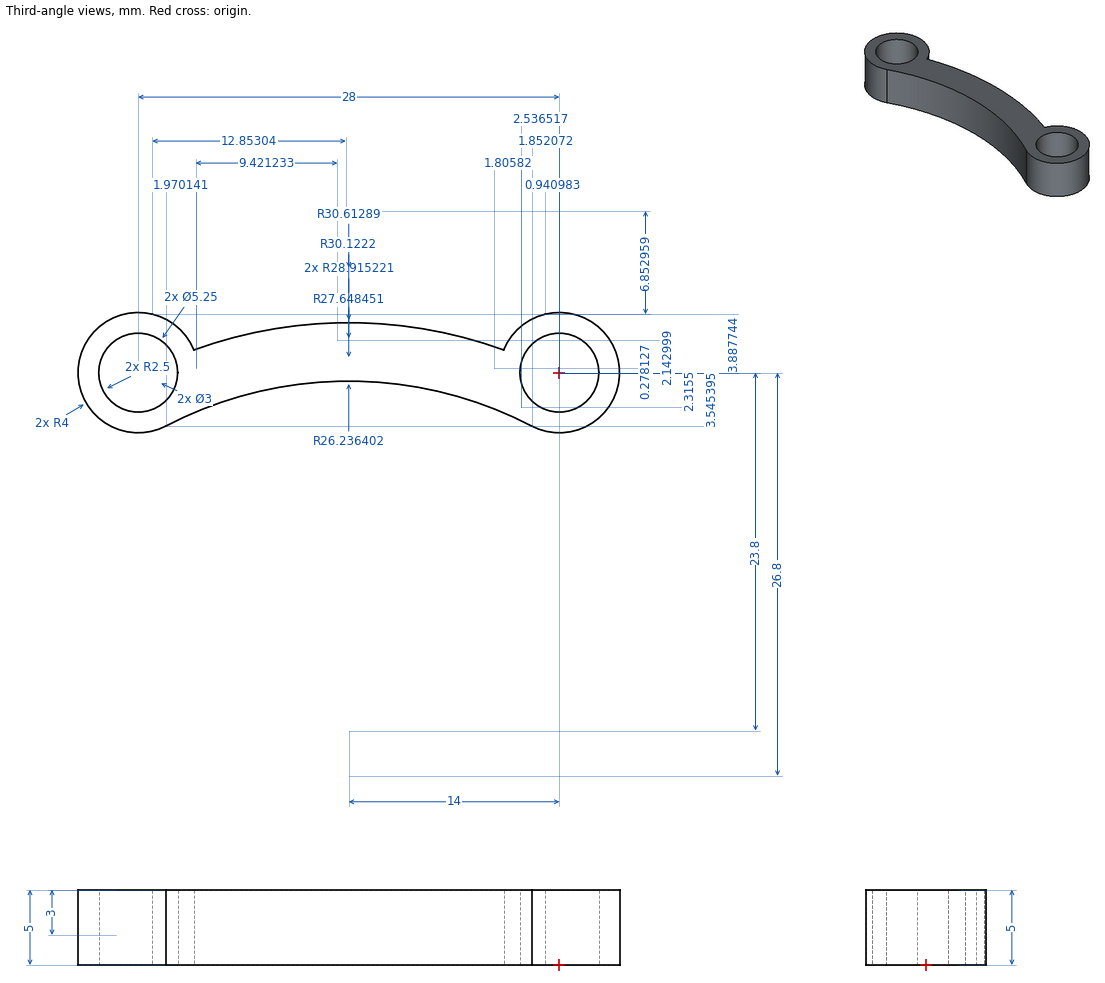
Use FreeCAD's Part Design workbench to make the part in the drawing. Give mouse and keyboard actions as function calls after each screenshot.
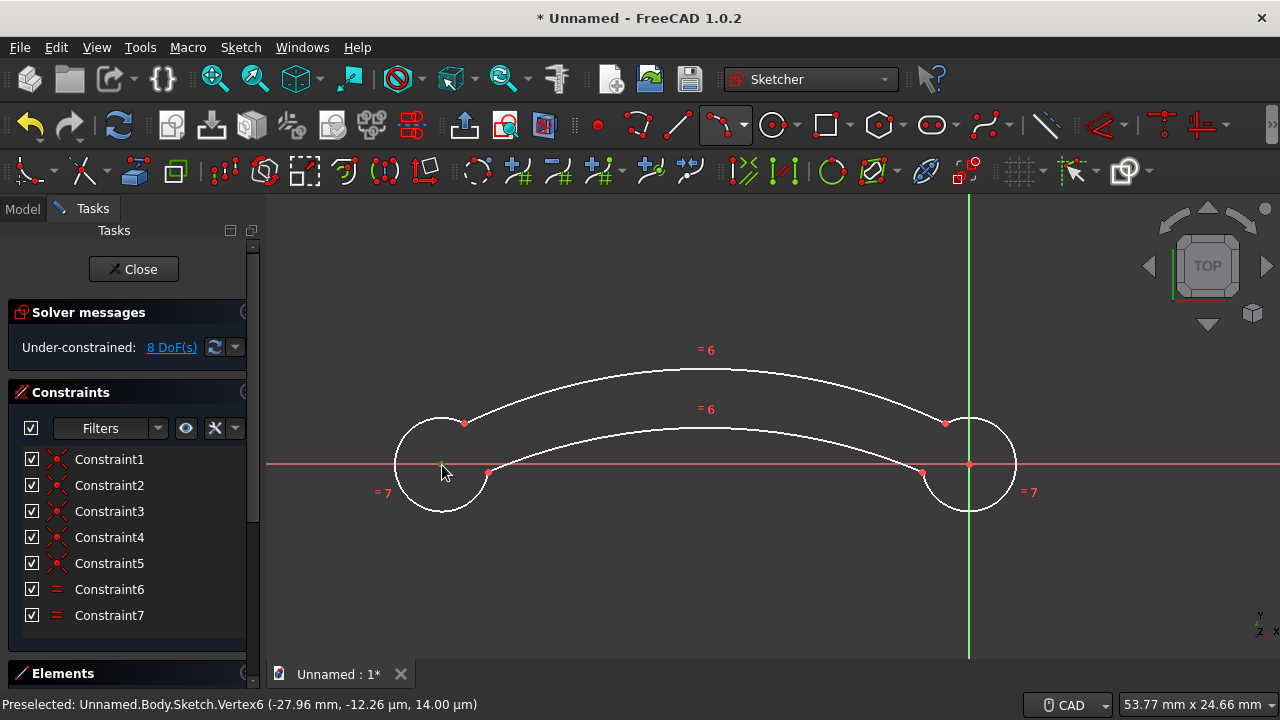
click(353, 464)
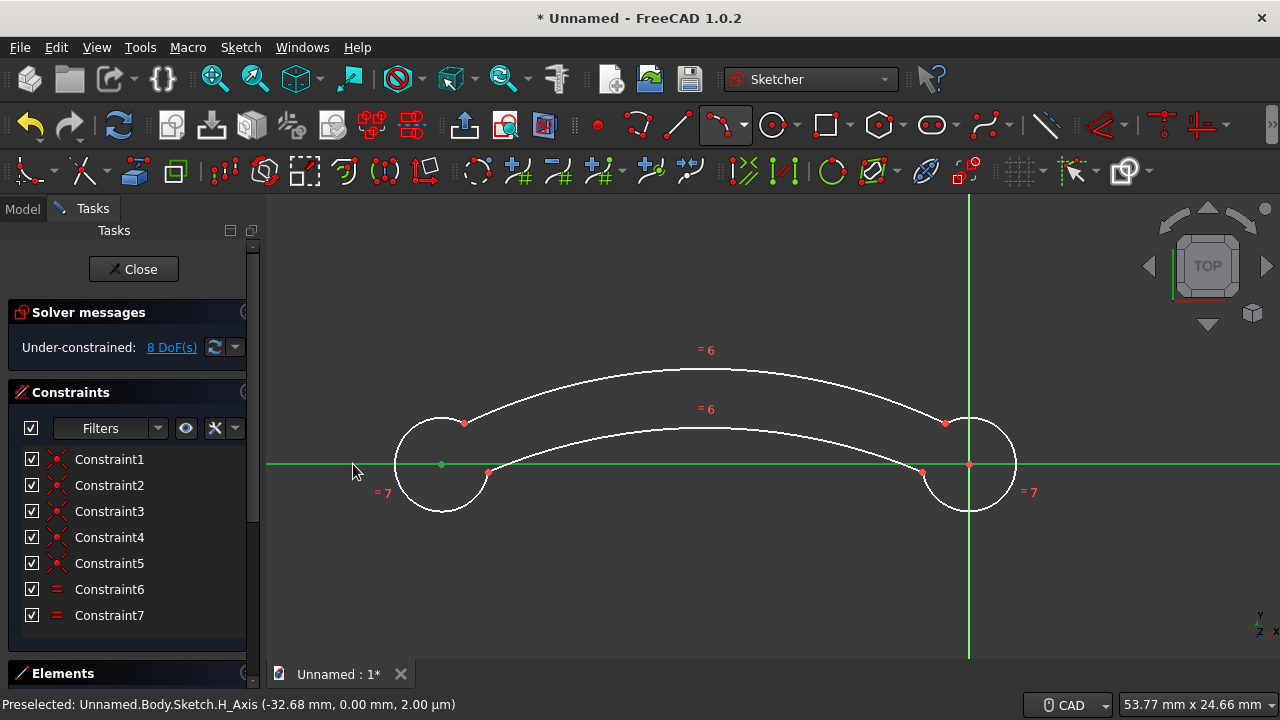
click(1162, 126)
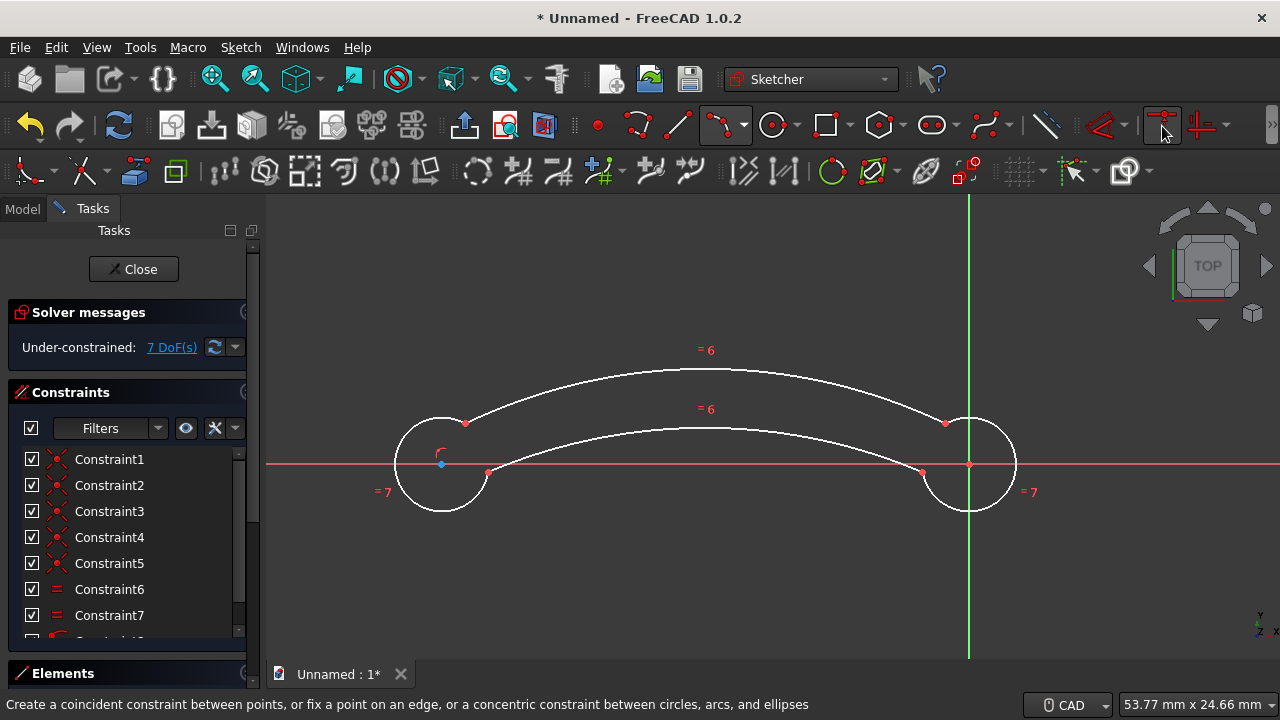
click(1100, 126)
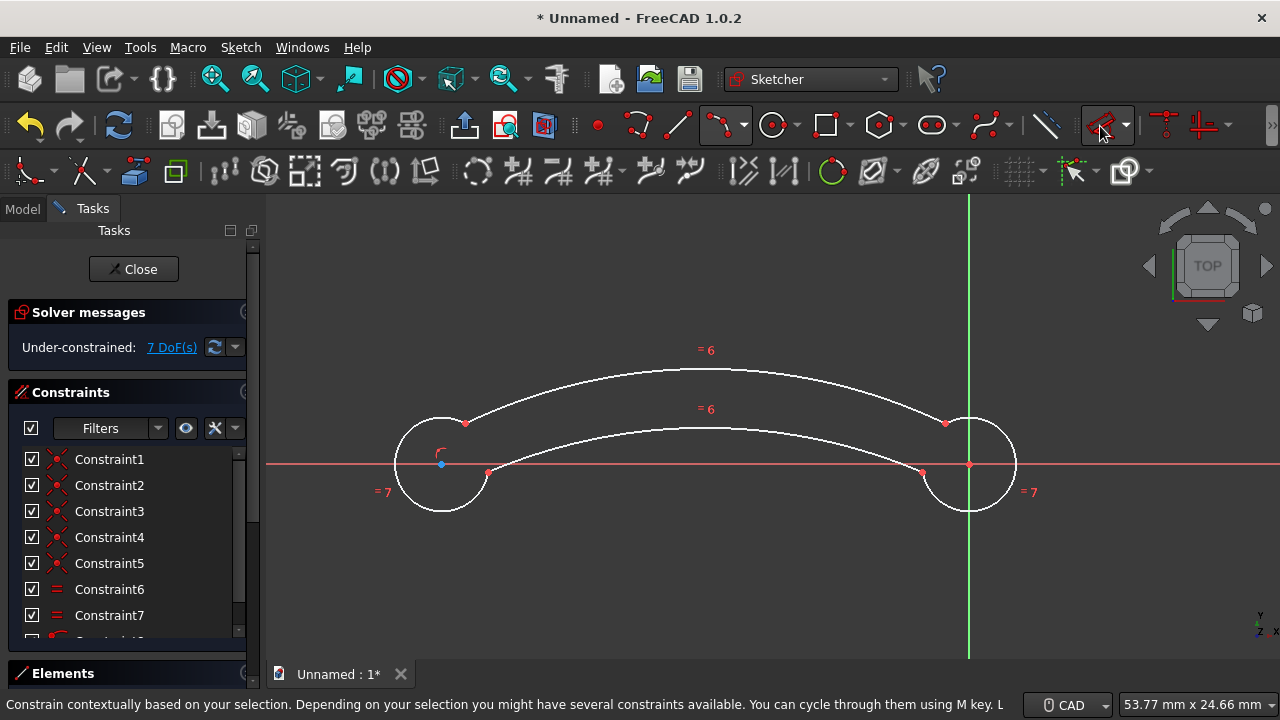
click(804, 378)
click(810, 347)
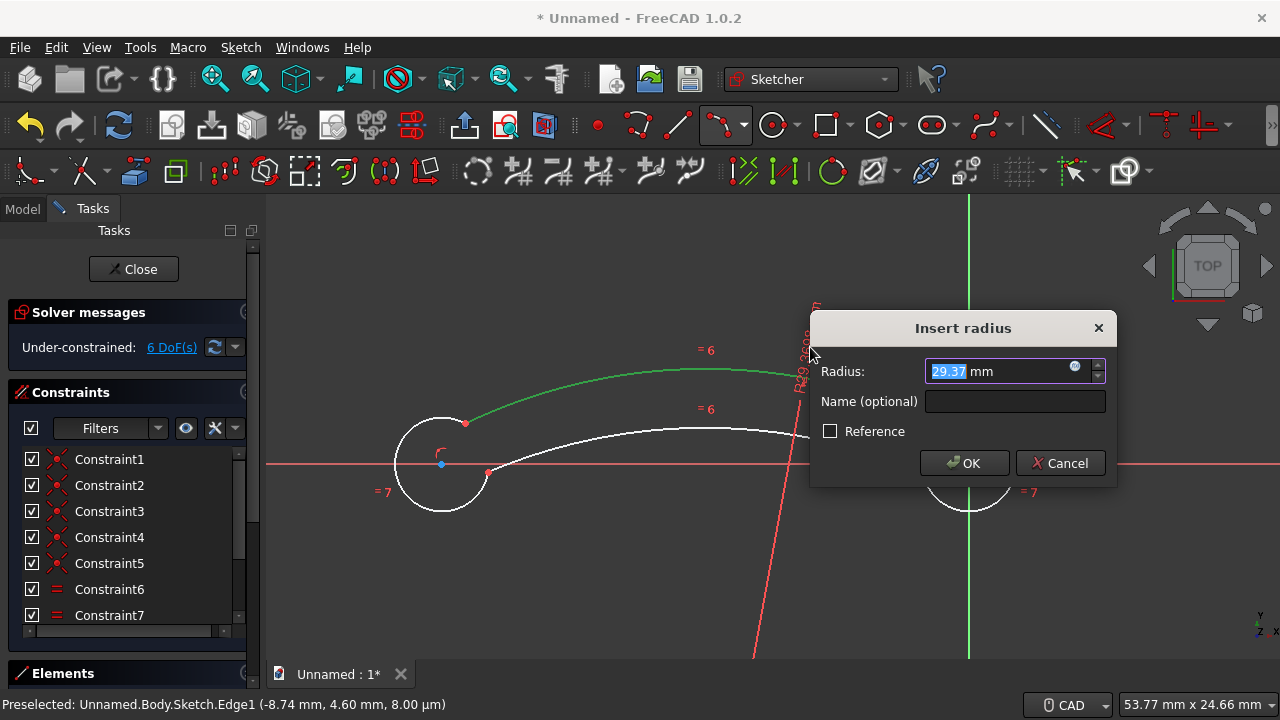
text(28.915221)
key(Return)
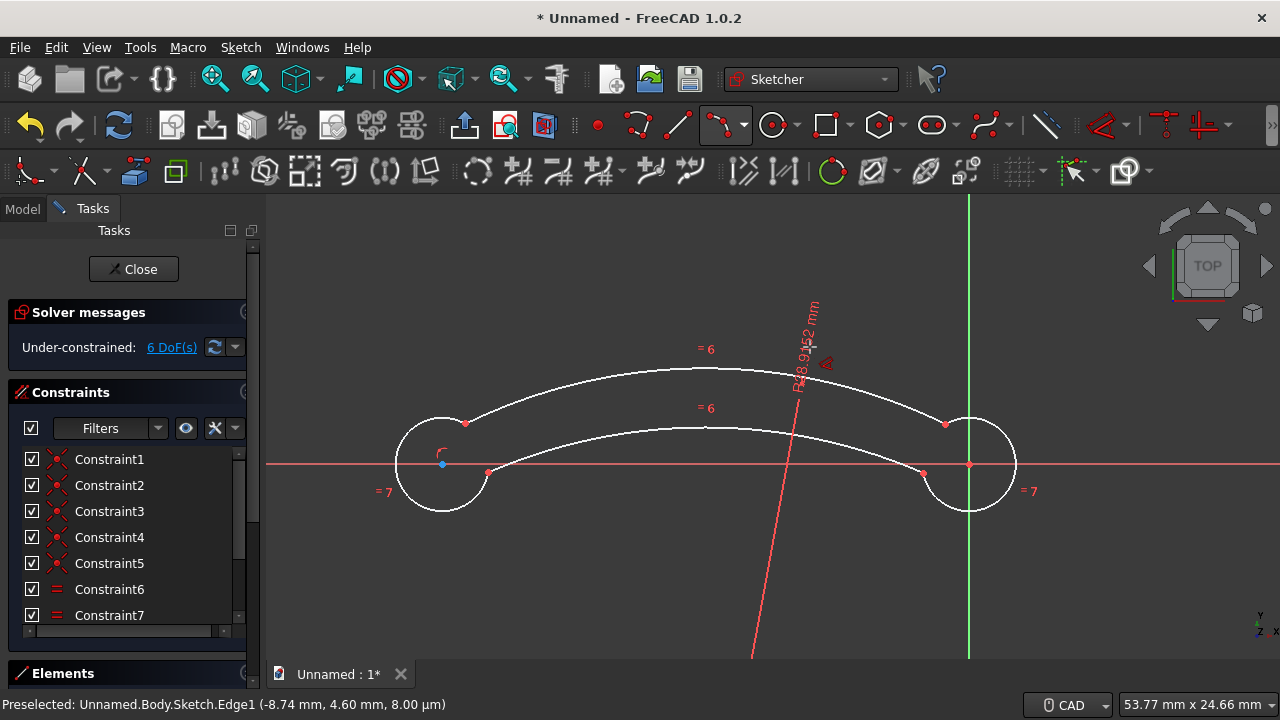
click(403, 439)
click(376, 422)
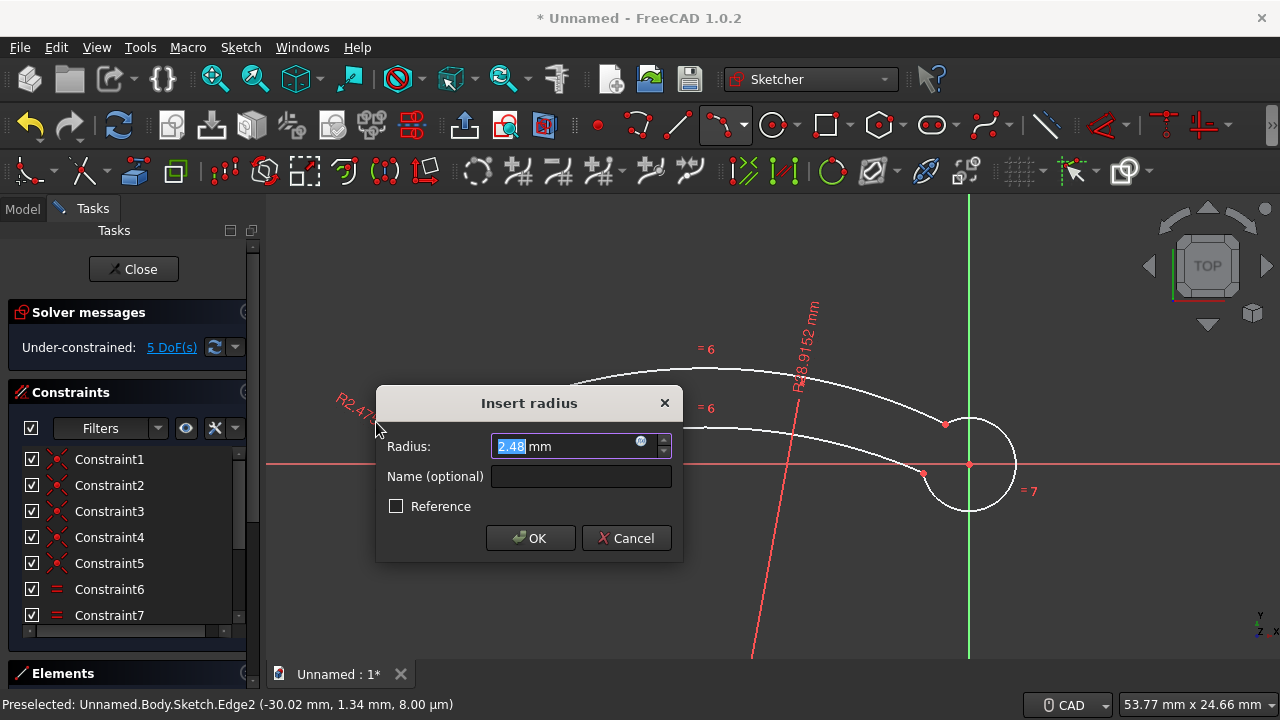
text(2.5)
key(Return)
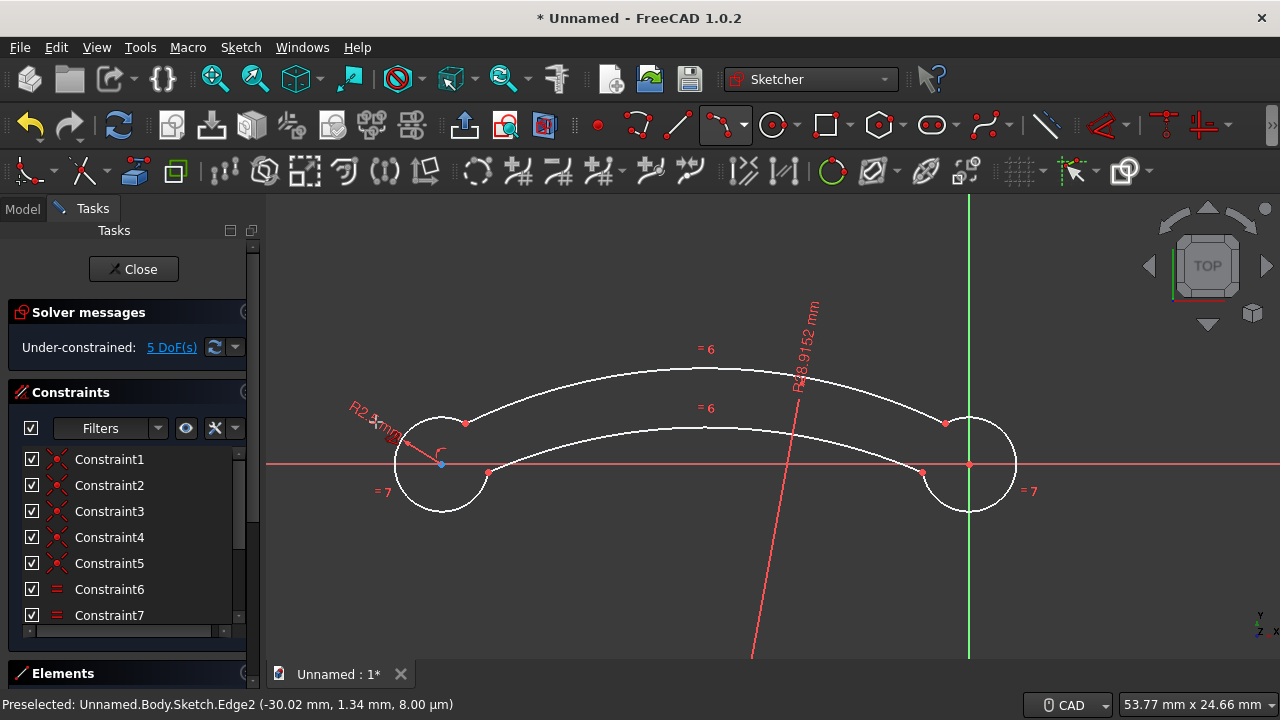
scroll(704, 222, down, 3)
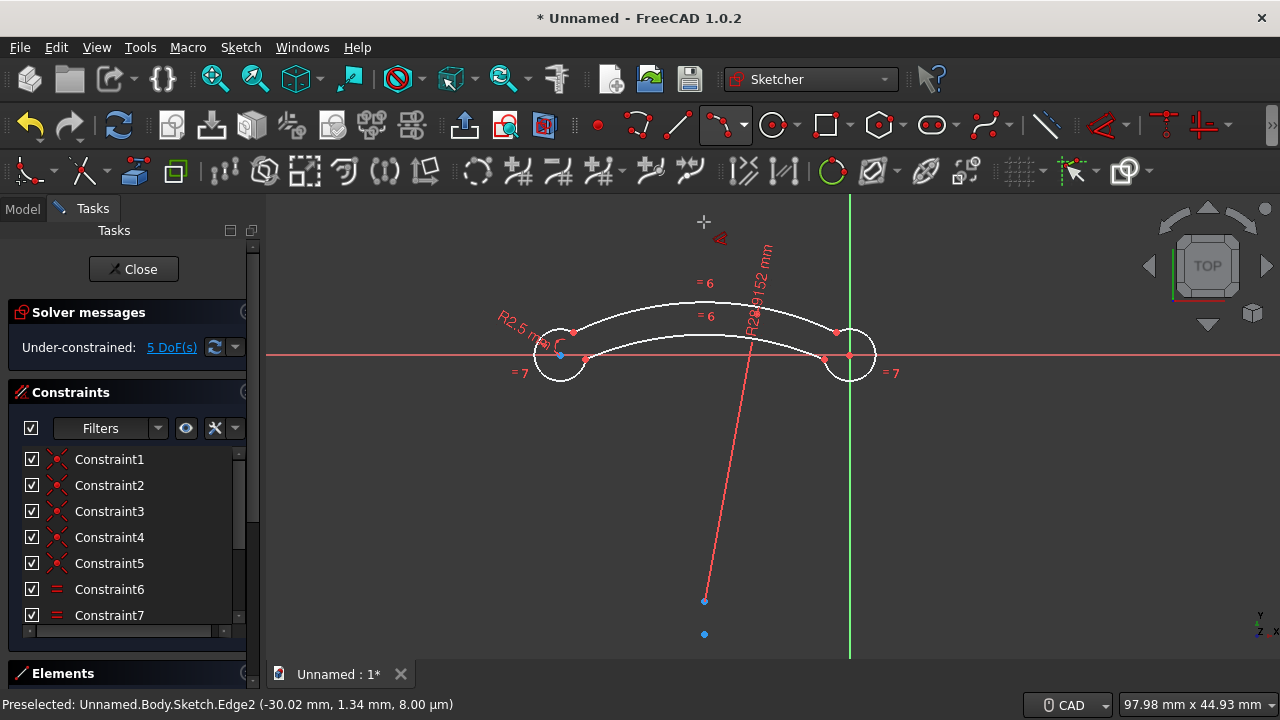
click(705, 602)
click(744, 321)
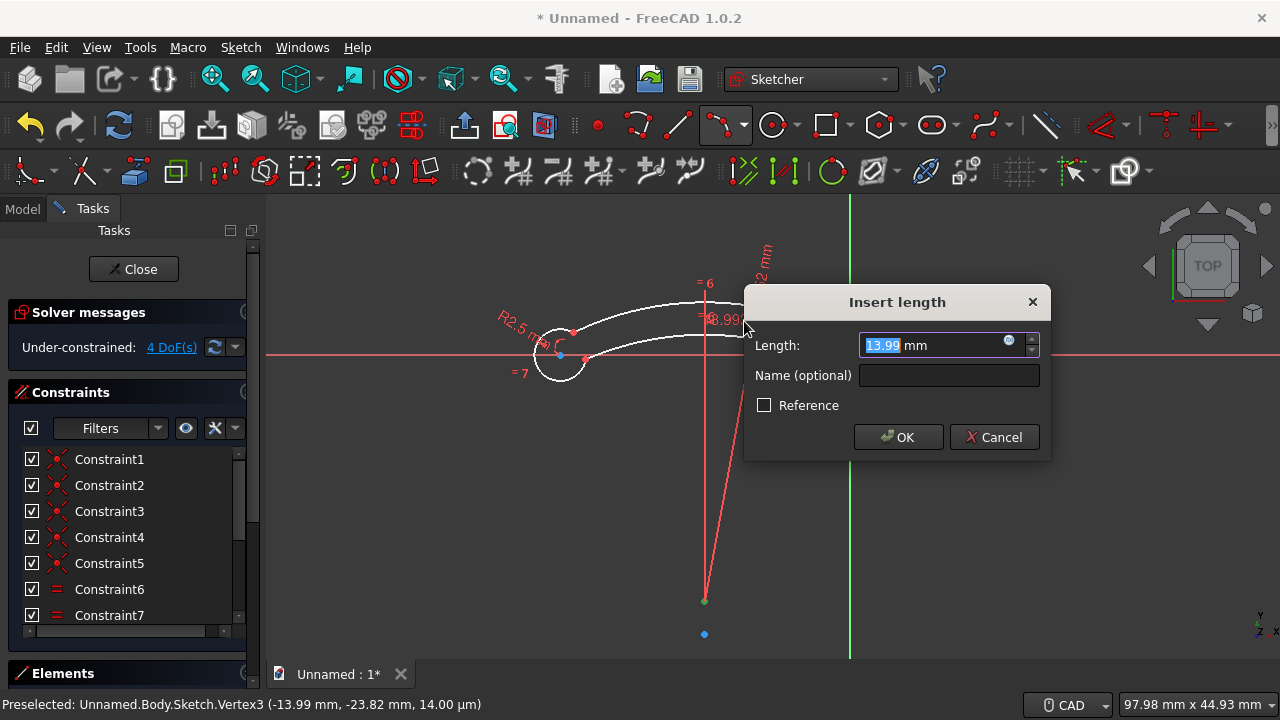
text(14)
key(Return)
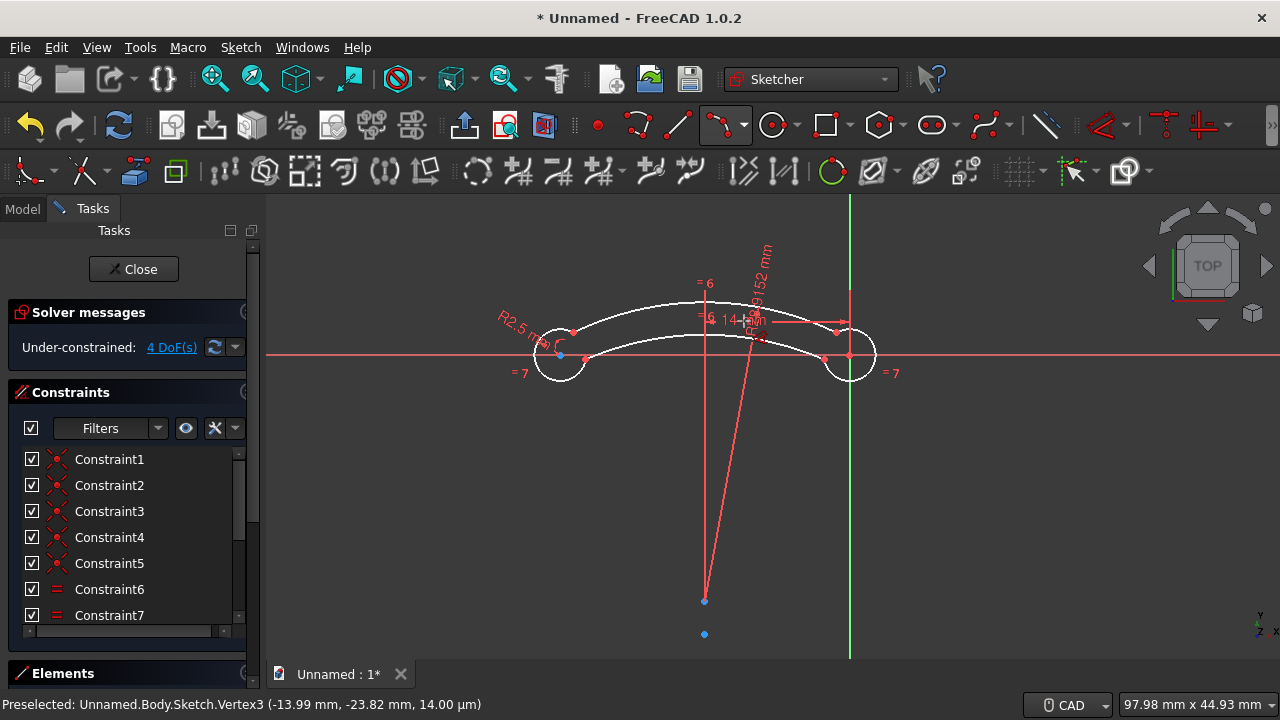
click(560, 355)
click(705, 389)